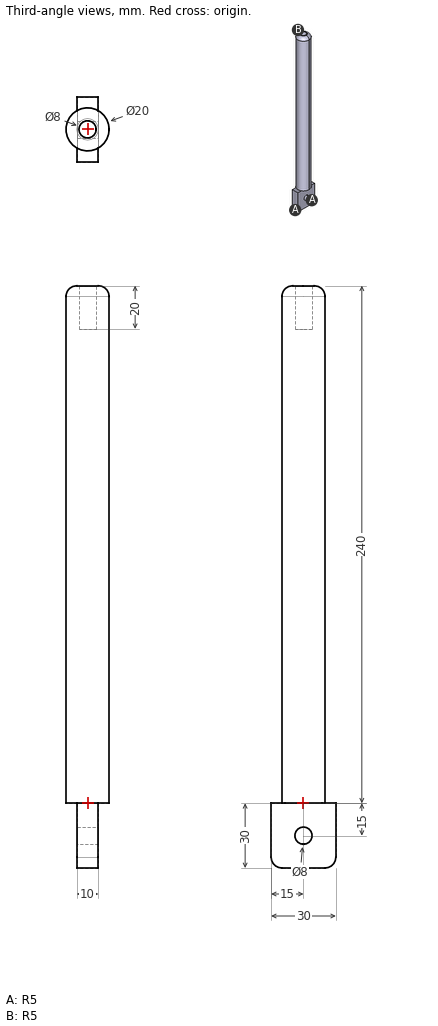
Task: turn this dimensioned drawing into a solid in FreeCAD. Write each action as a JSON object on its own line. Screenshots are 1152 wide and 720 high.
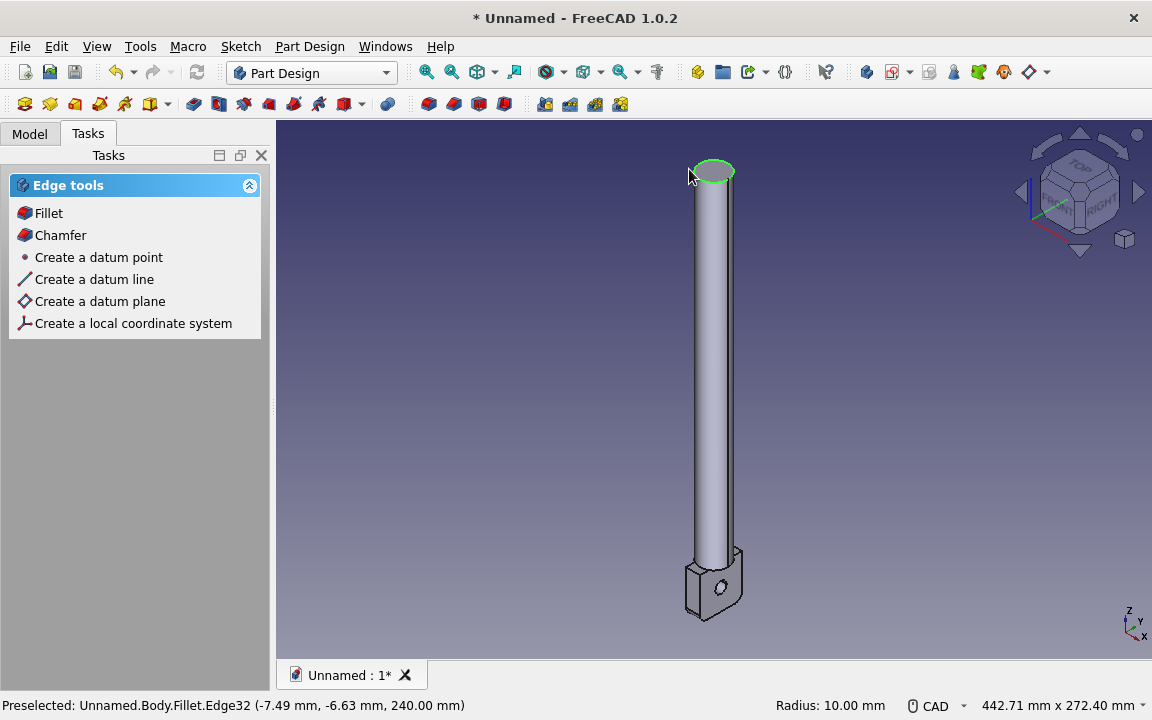
{"action": "left_click", "coordinate": [429, 104]}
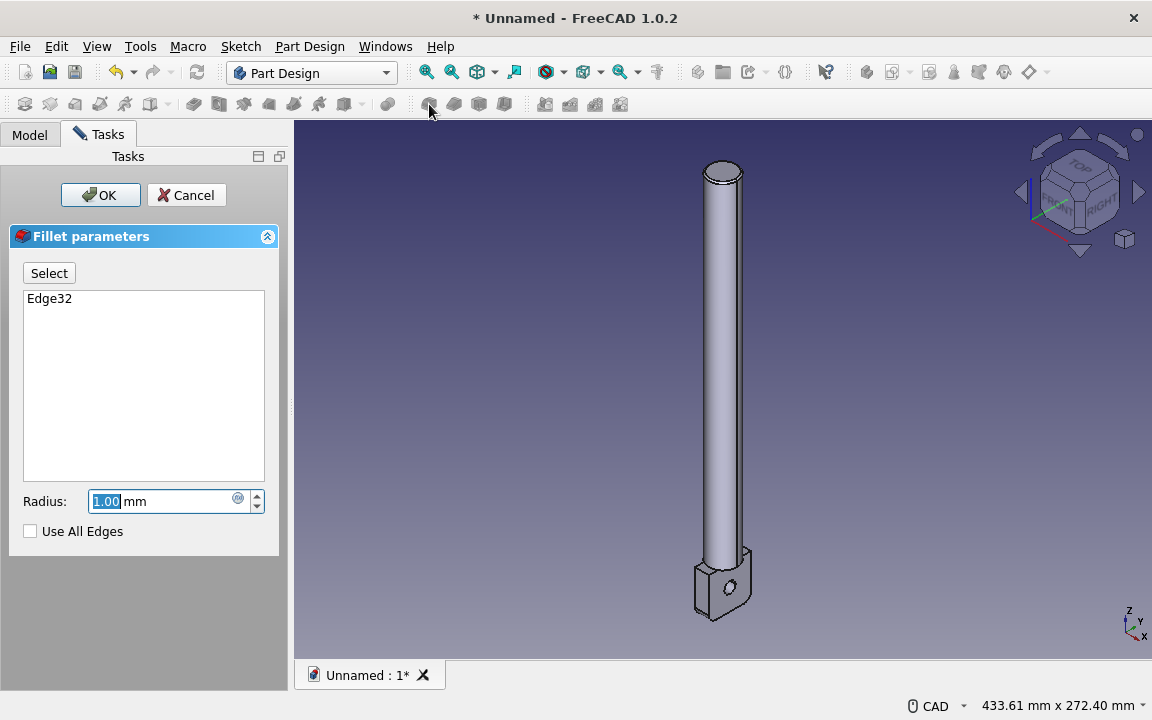
{"action": "type", "text": "5"}
{"action": "key", "text": "Tab"}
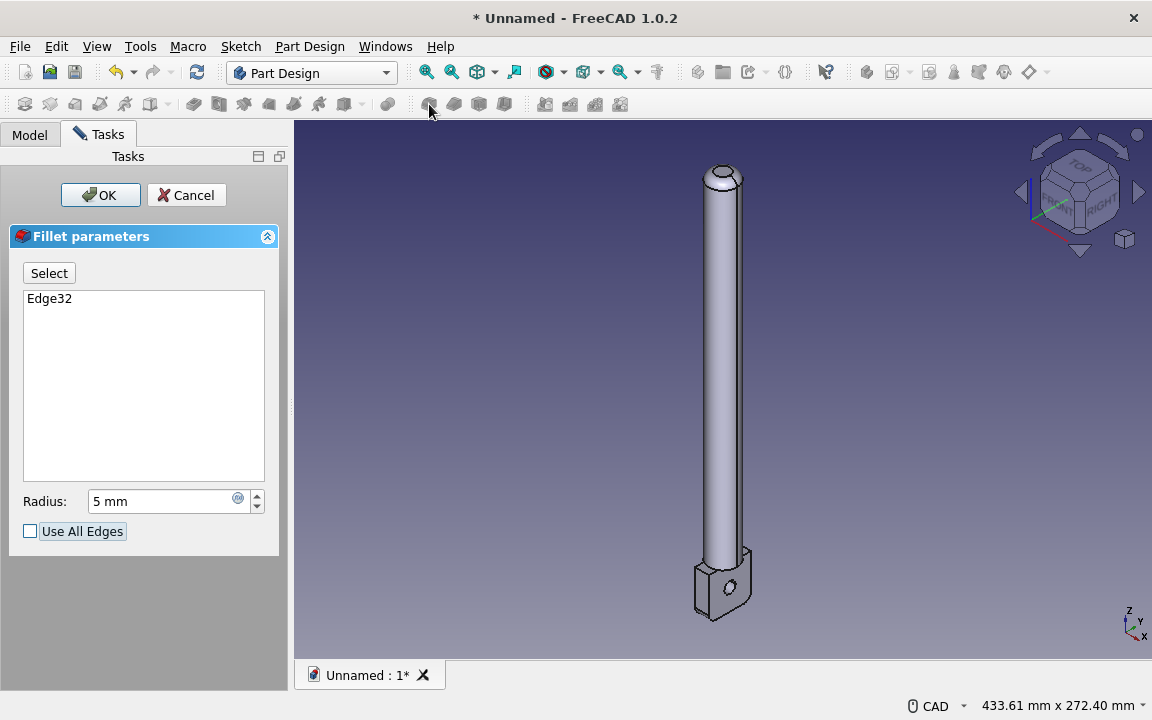
{"action": "left_click", "coordinate": [101, 195]}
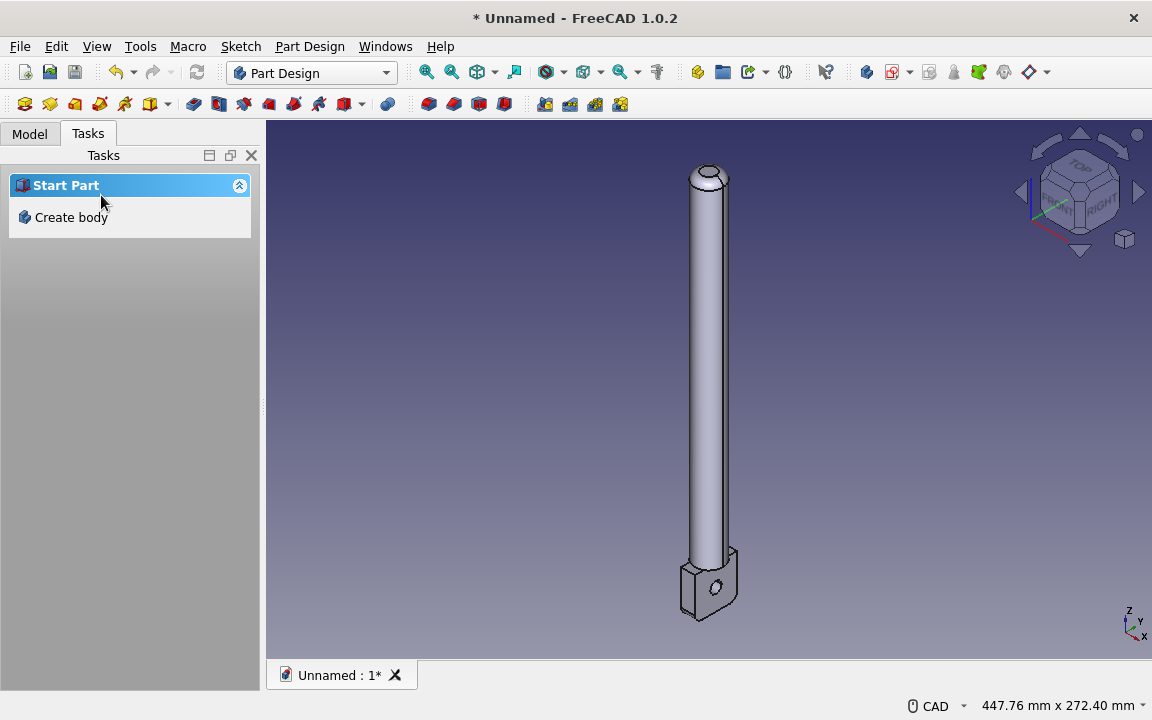
{"action": "key", "text": "2"}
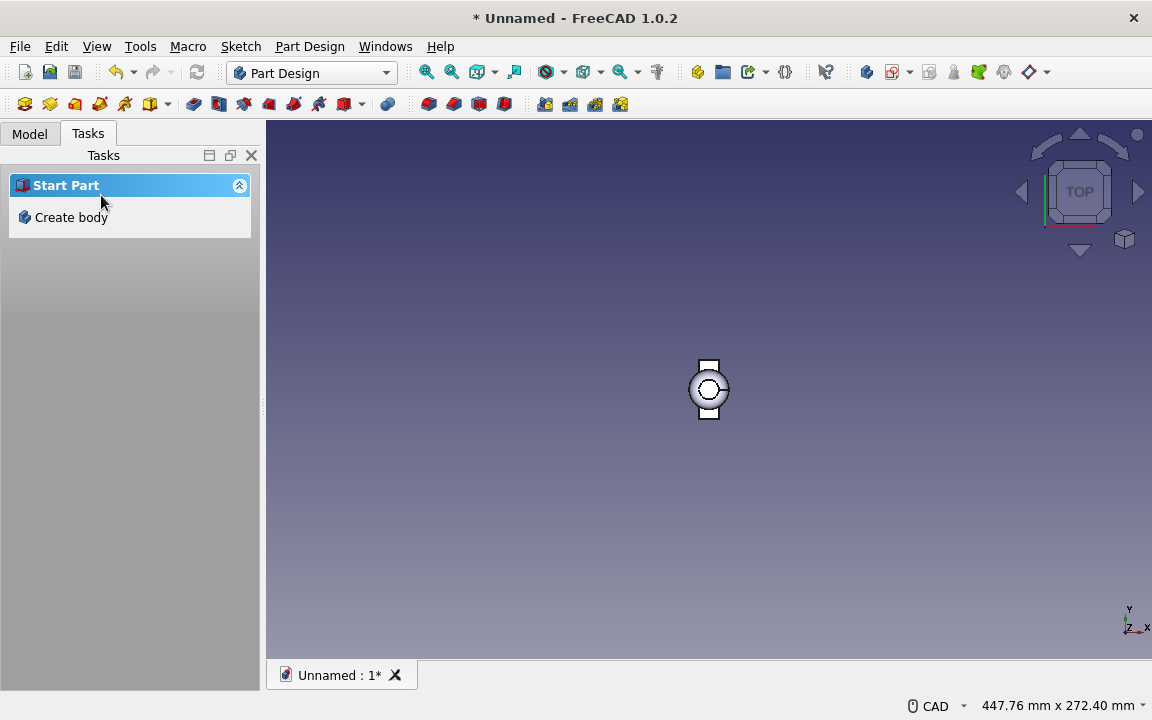
{"action": "left_click", "coordinate": [427, 72]}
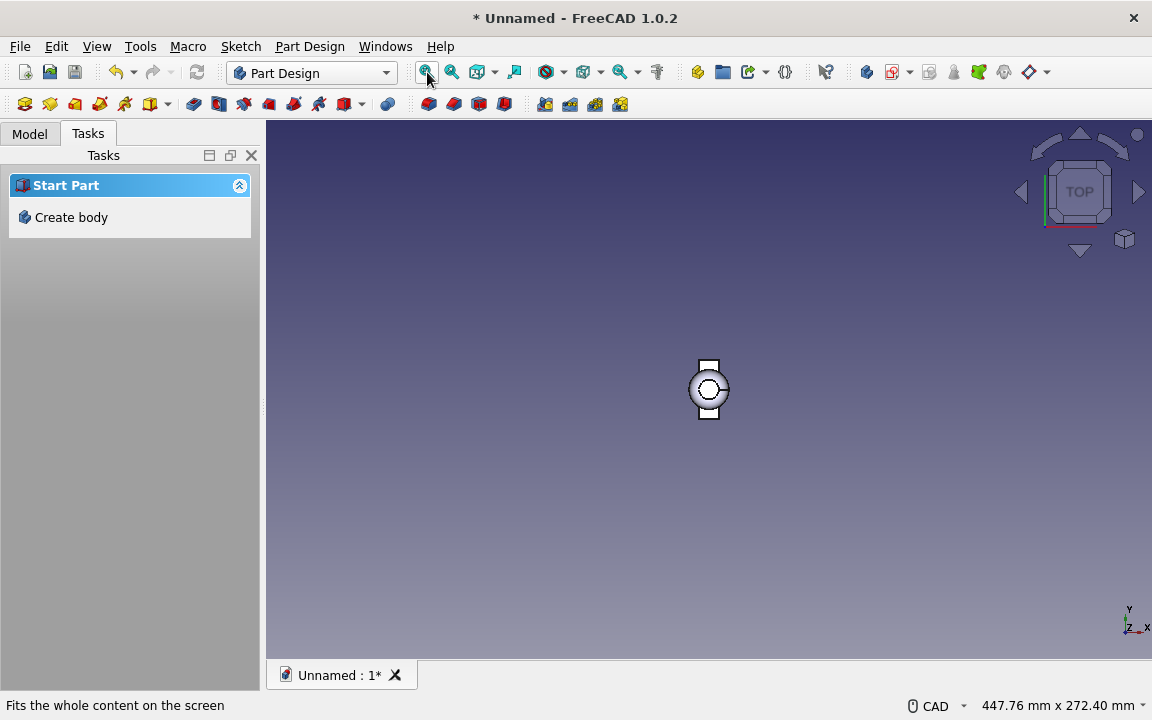
{"action": "left_click", "coordinate": [709, 388]}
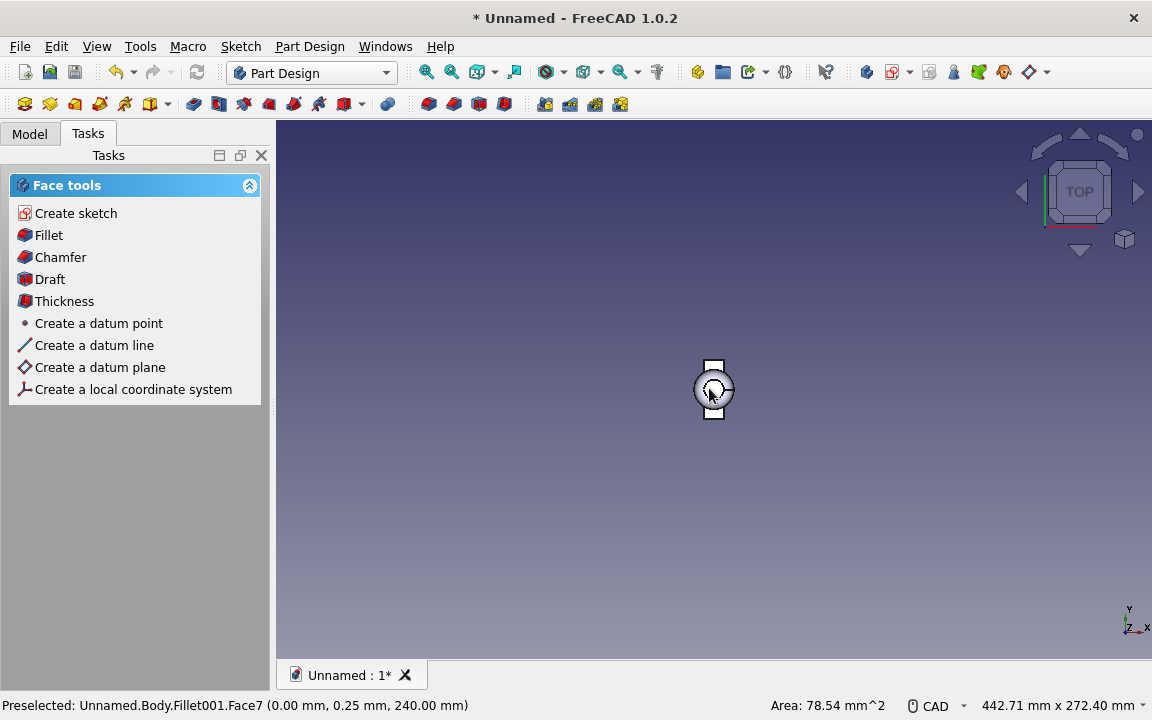
{"action": "left_click", "coordinate": [892, 72]}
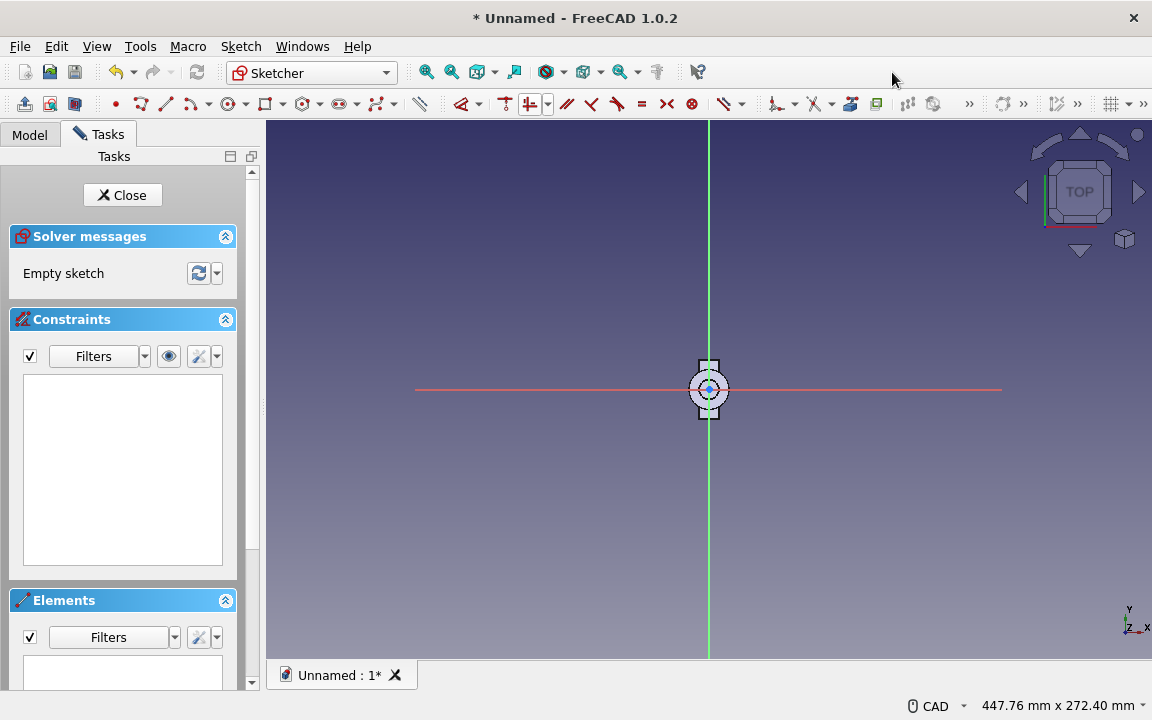
{"action": "scroll", "coordinate": [713, 390], "scroll_direction": "up", "scroll_amount": 15}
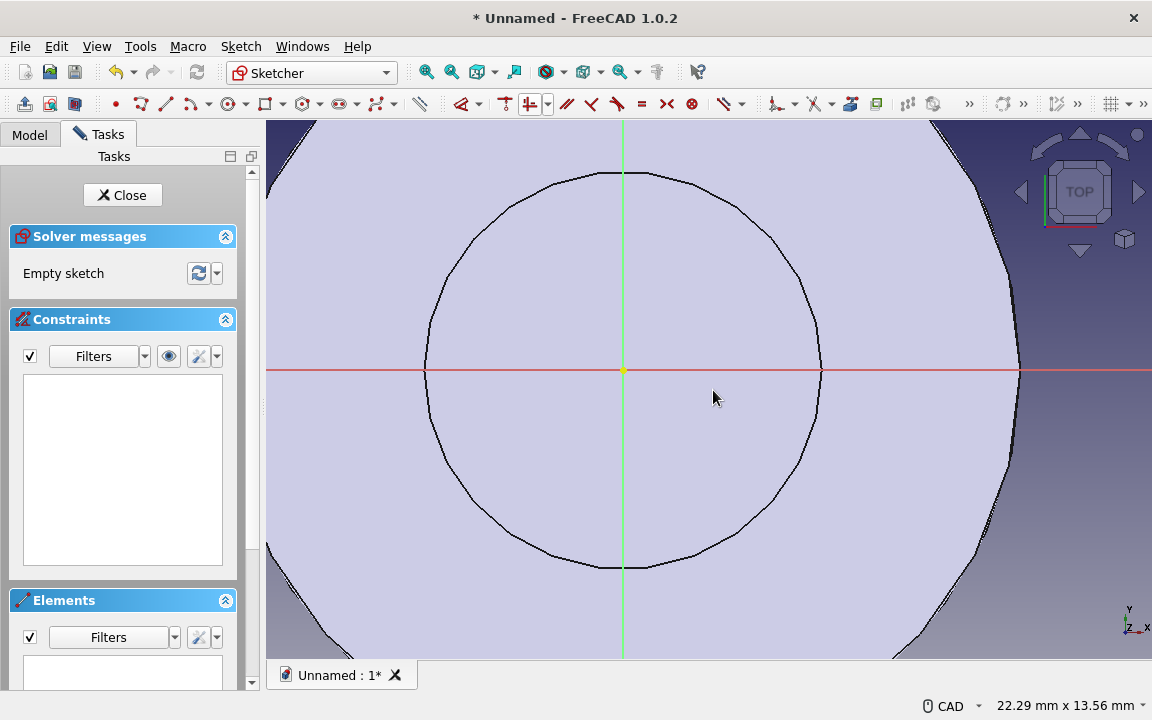
{"action": "key", "text": "g c"}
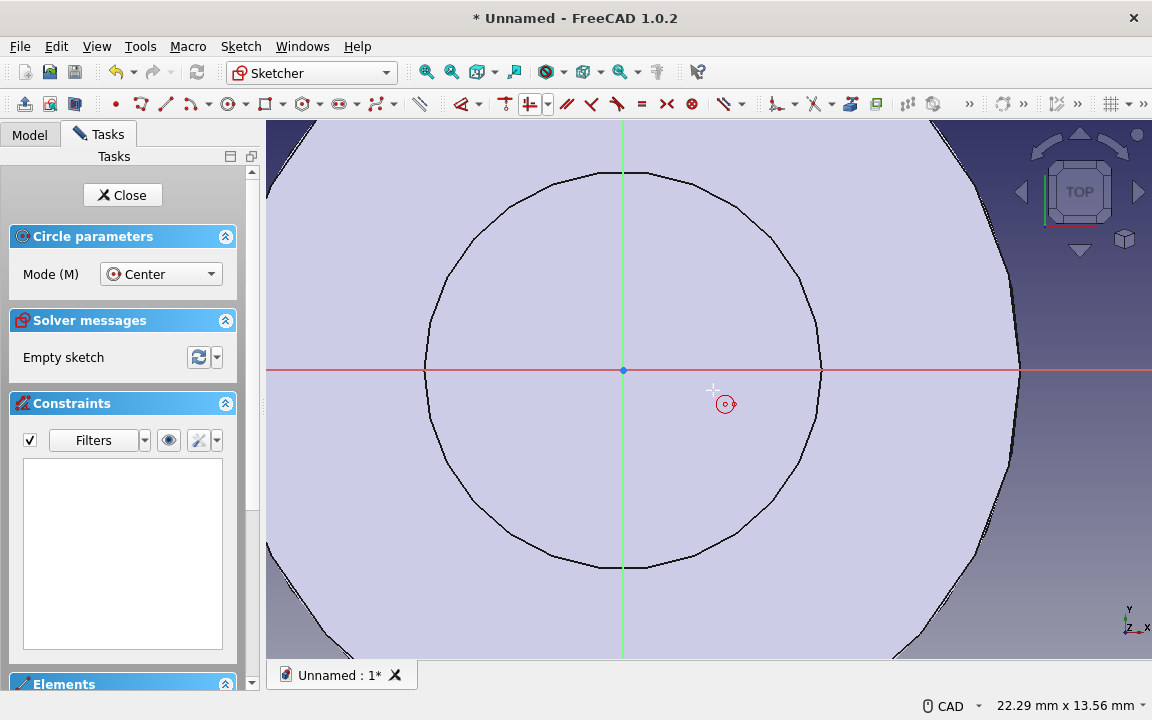
{"action": "left_click", "coordinate": [623, 370]}
{"action": "left_click", "coordinate": [735, 258]}
{"action": "key", "text": "Escape"}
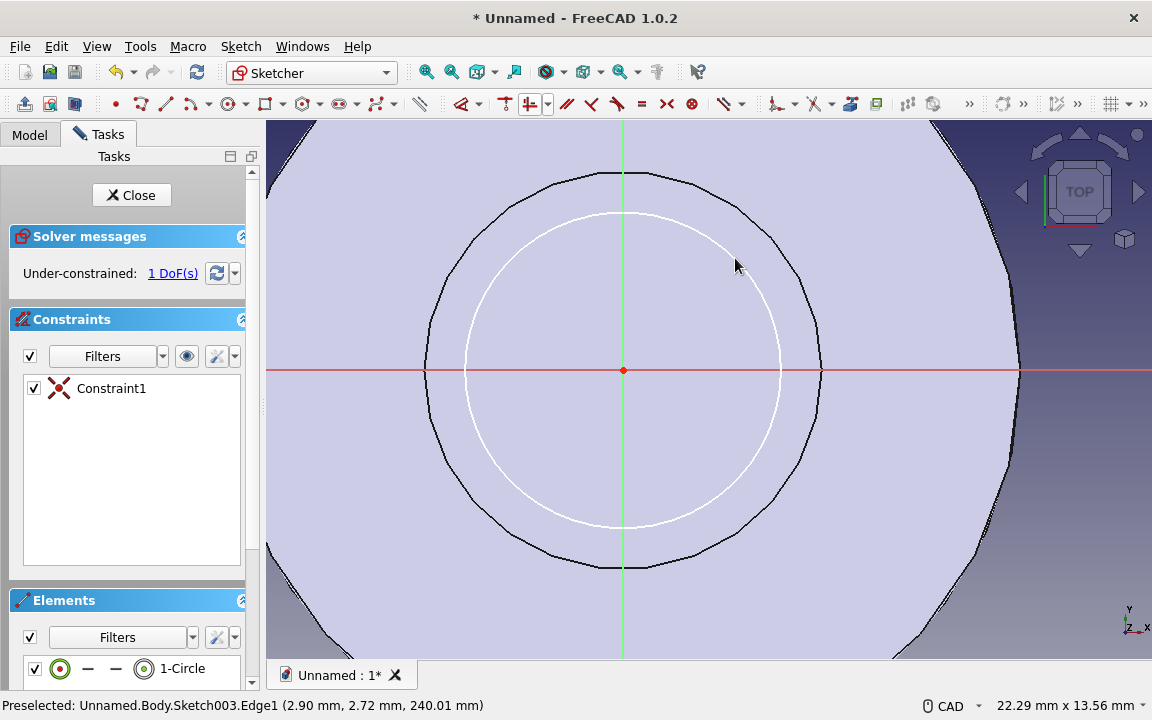
{"action": "key", "text": "d"}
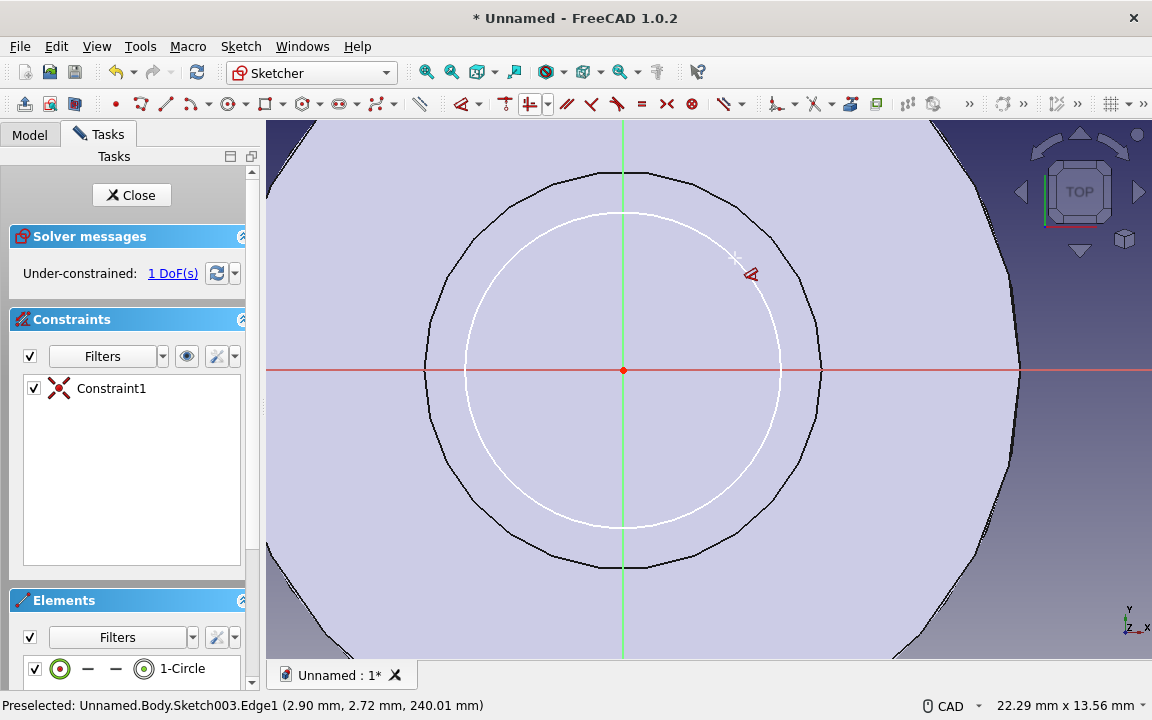
{"action": "left_click", "coordinate": [734, 258]}
{"action": "left_click", "coordinate": [756, 235]}